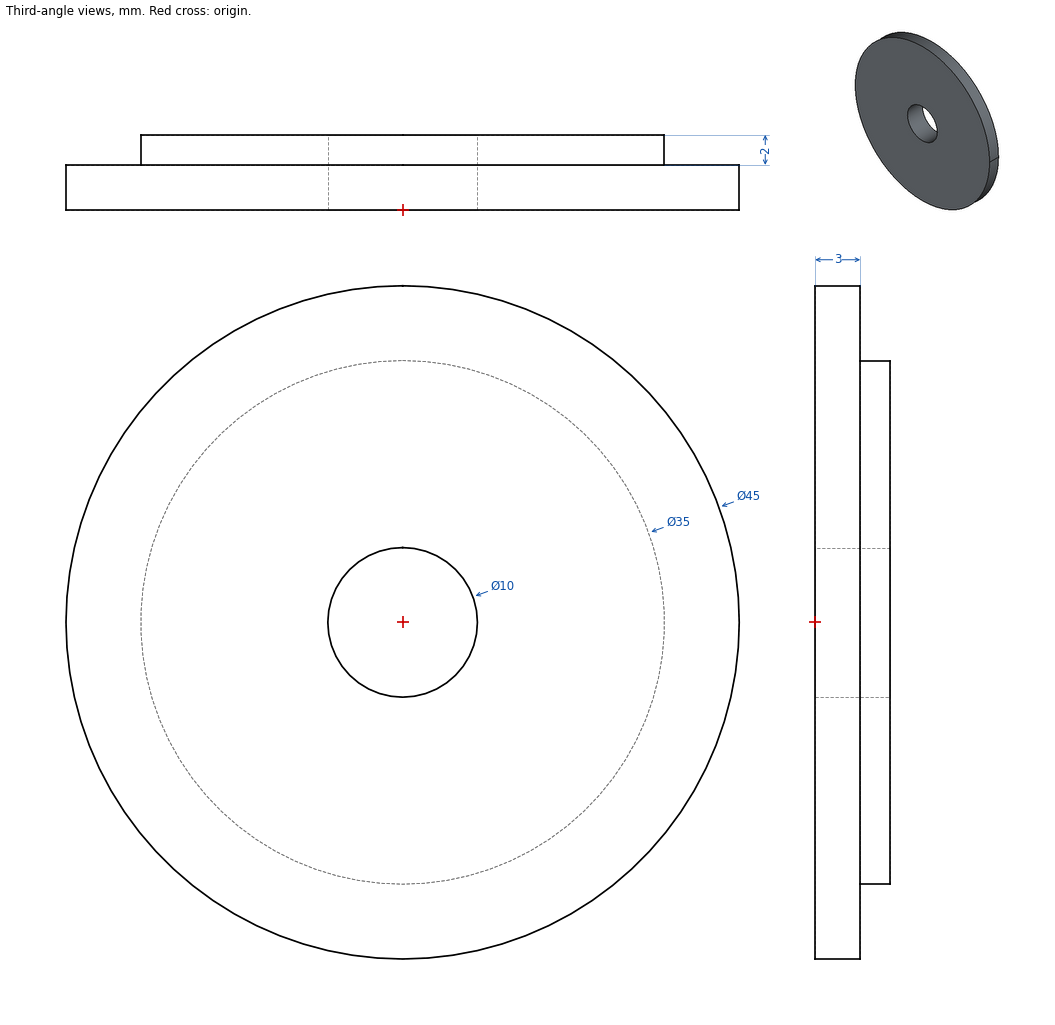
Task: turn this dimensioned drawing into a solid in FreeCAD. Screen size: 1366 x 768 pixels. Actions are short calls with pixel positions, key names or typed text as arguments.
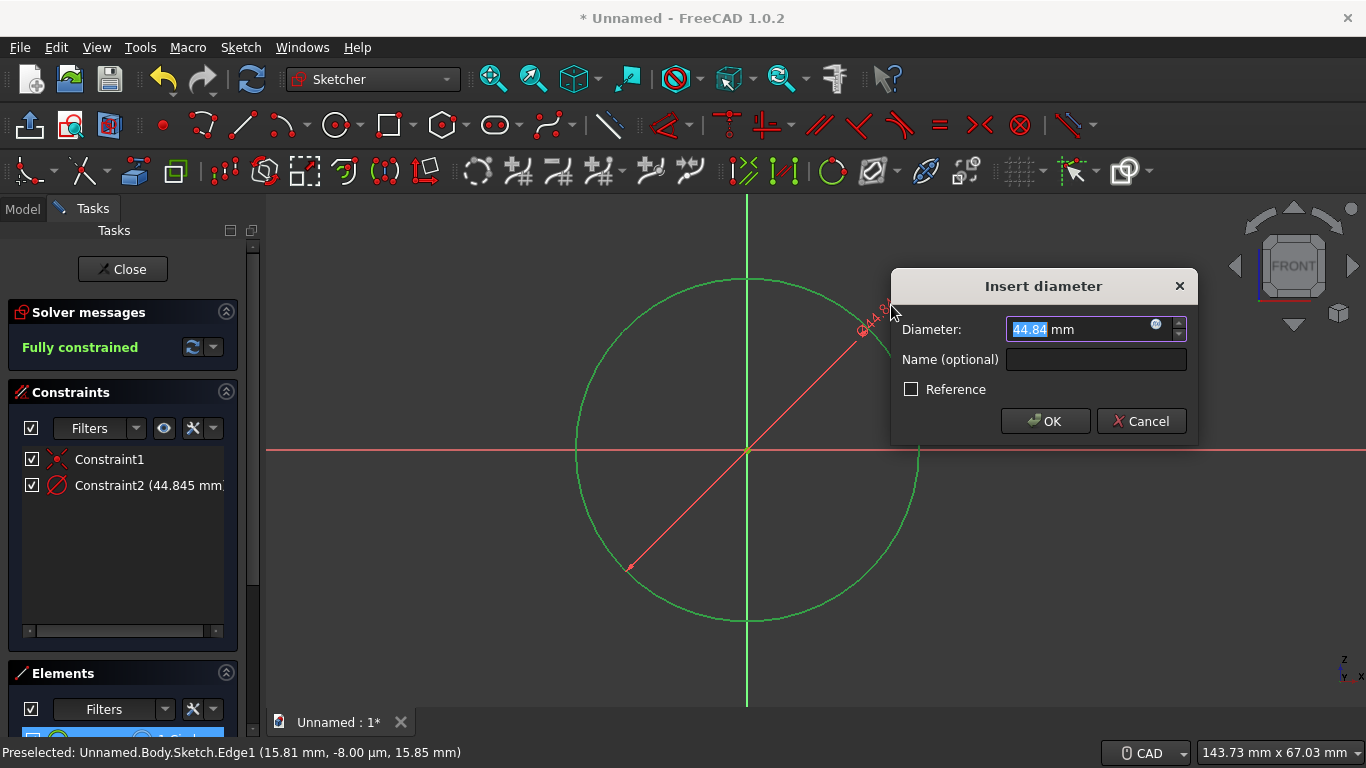
text(45)
key(Return)
key(Escape)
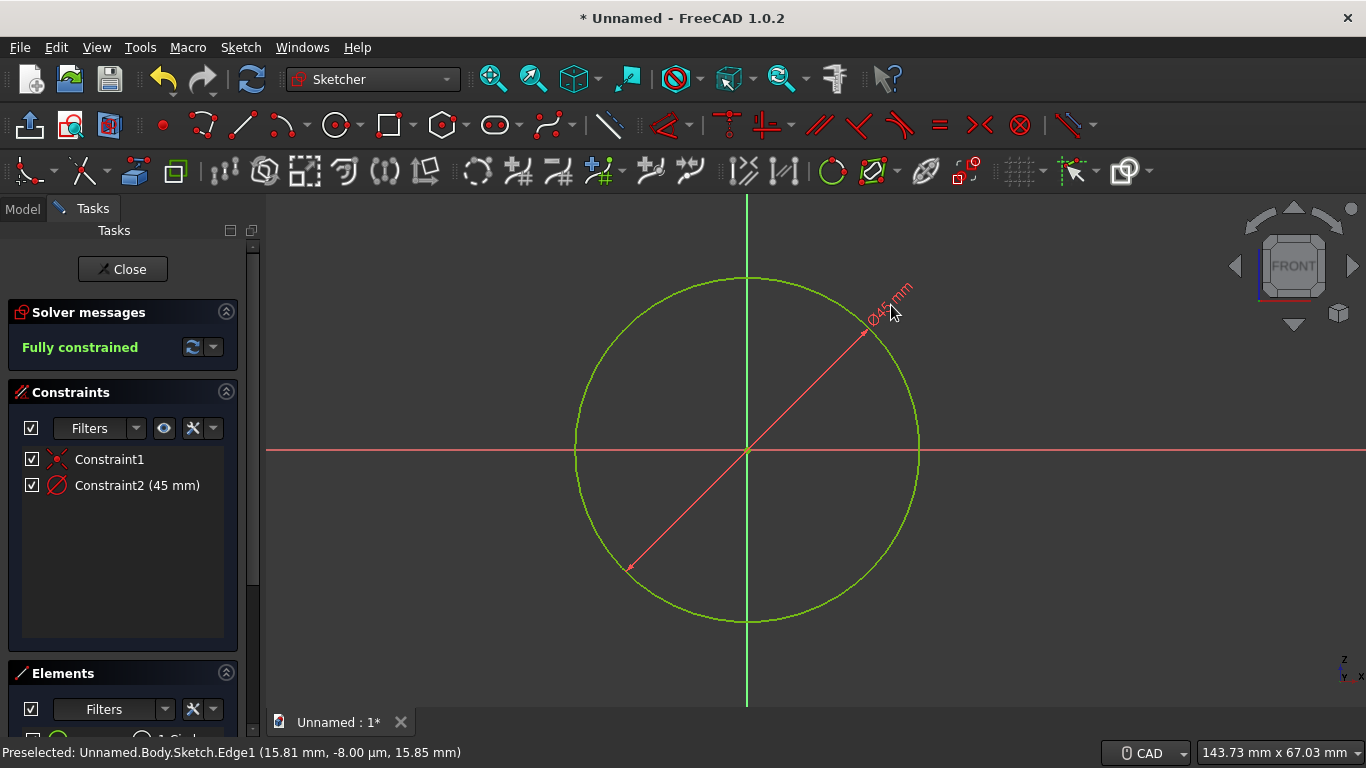
click(123, 269)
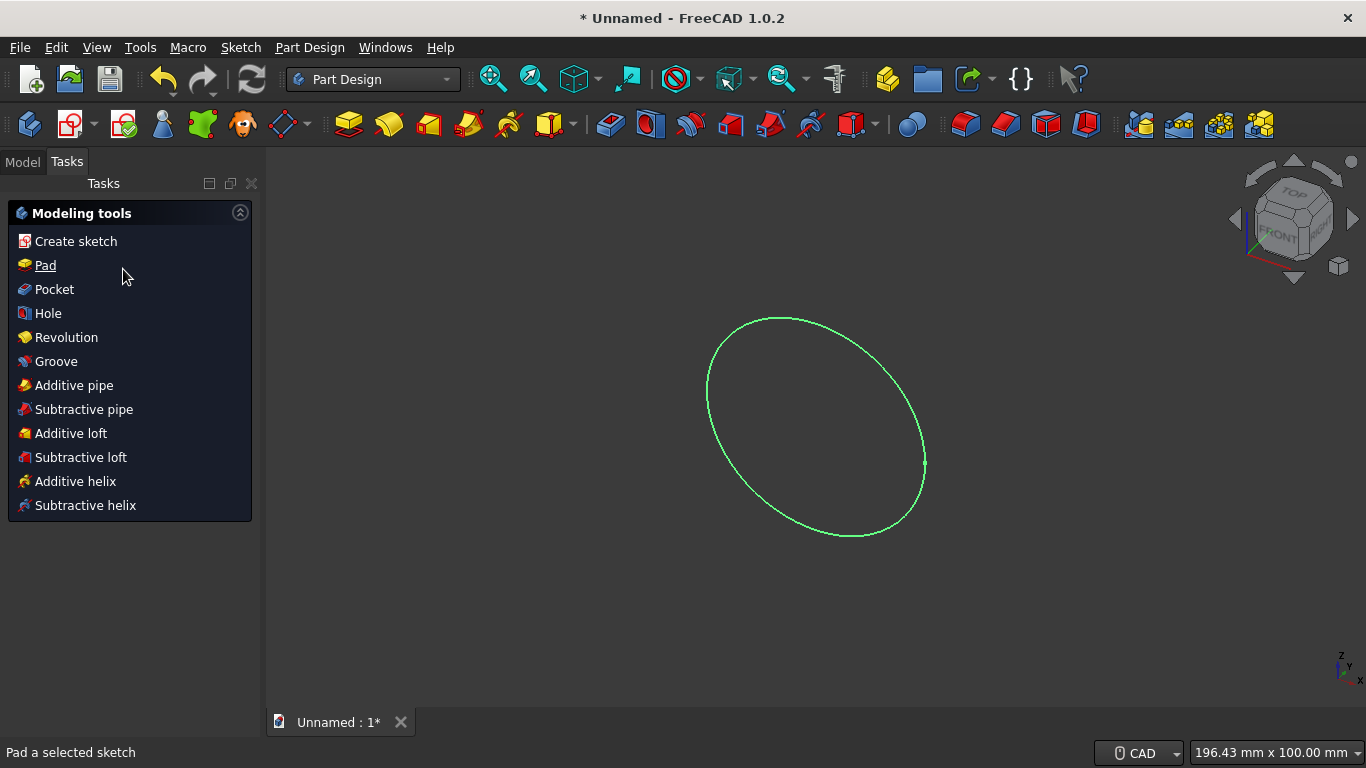
click(350, 124)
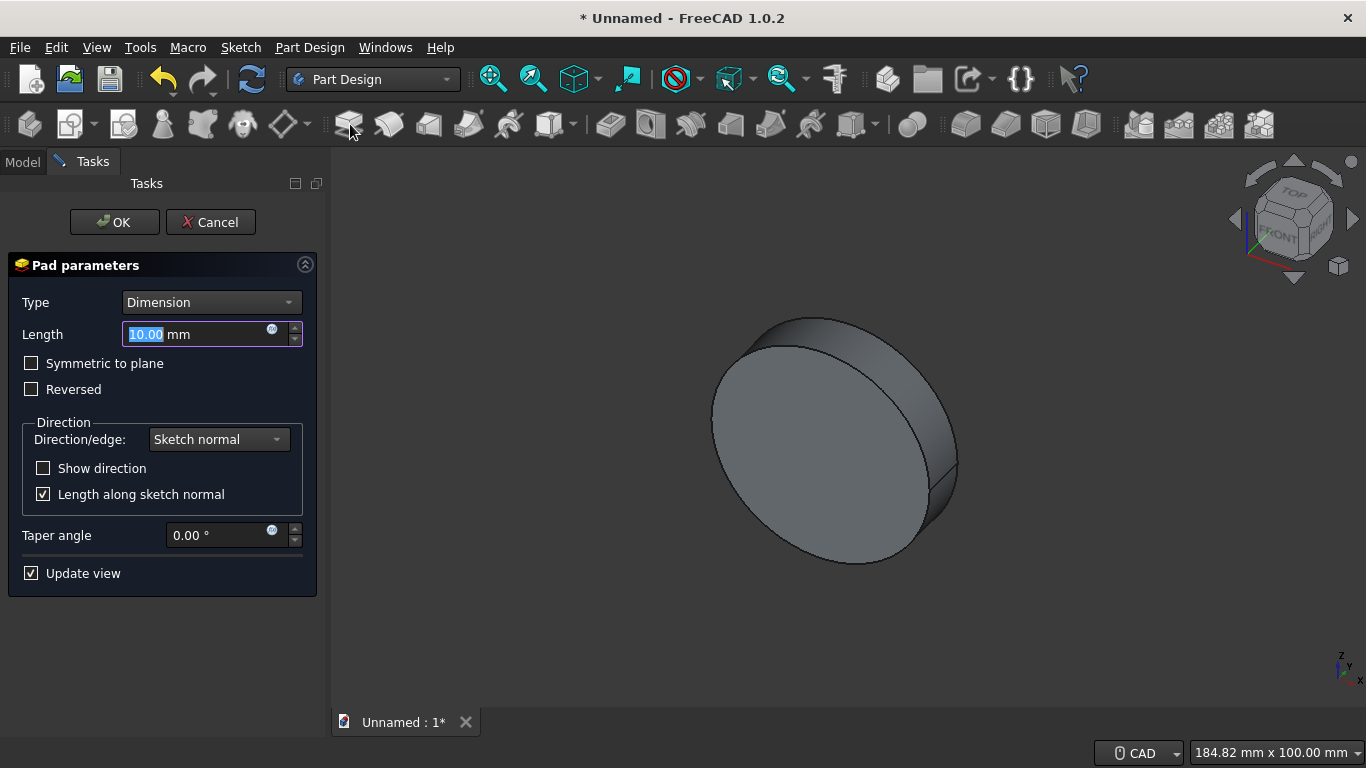
text(3)
key(Tab)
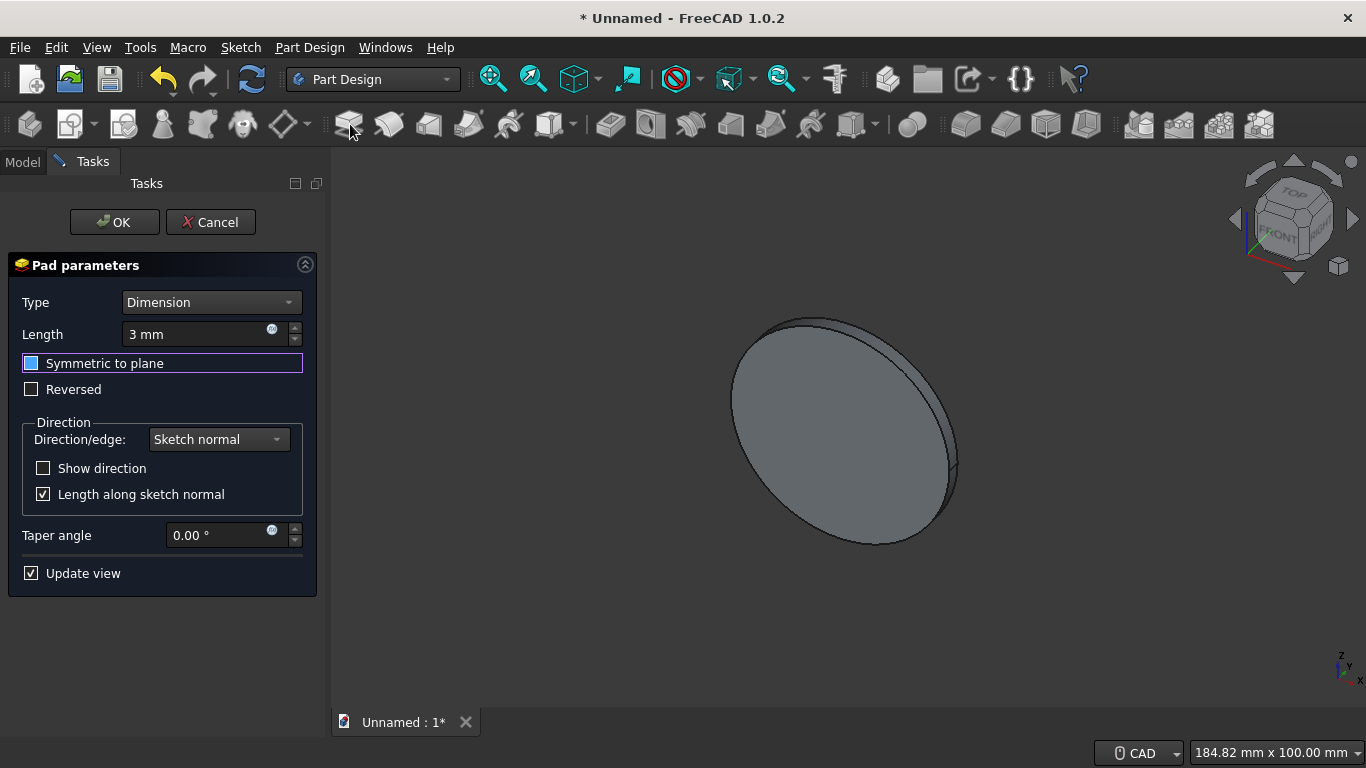
click(30, 389)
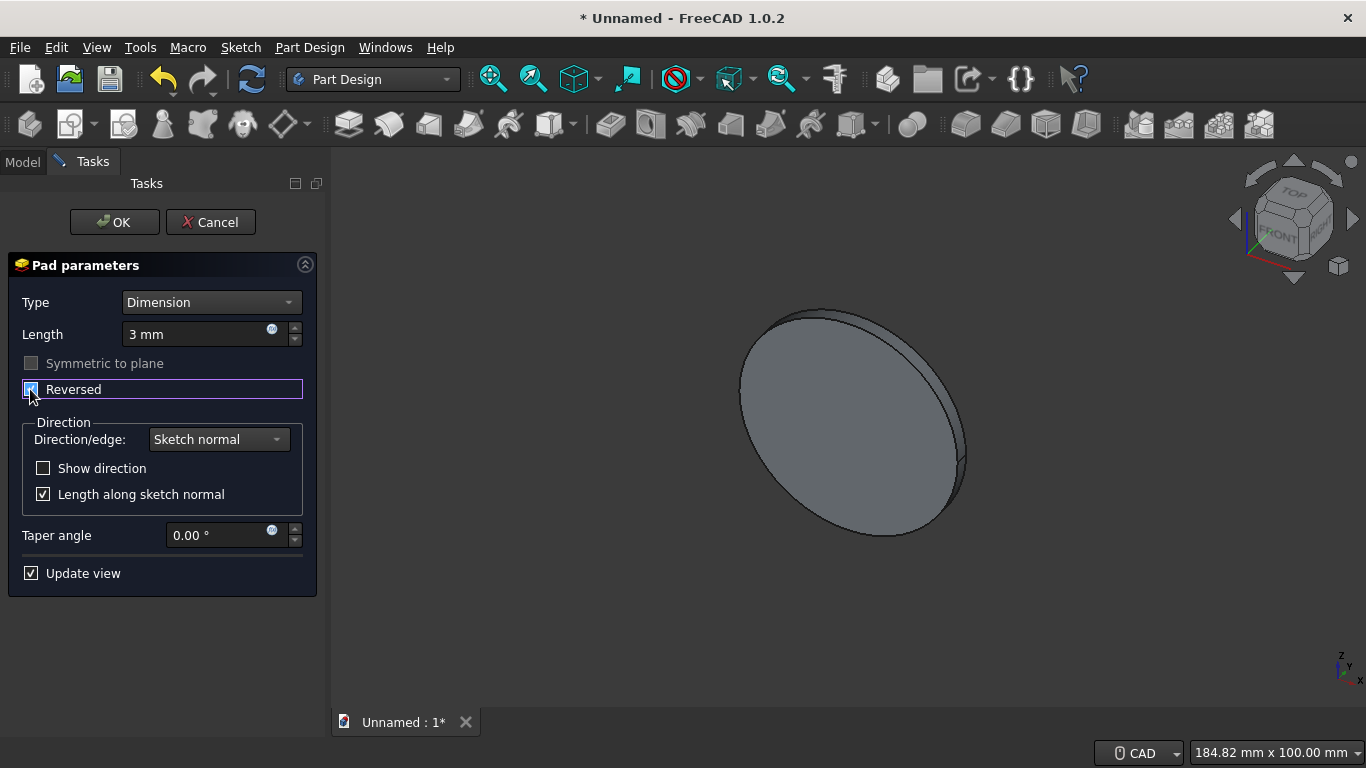
click(115, 222)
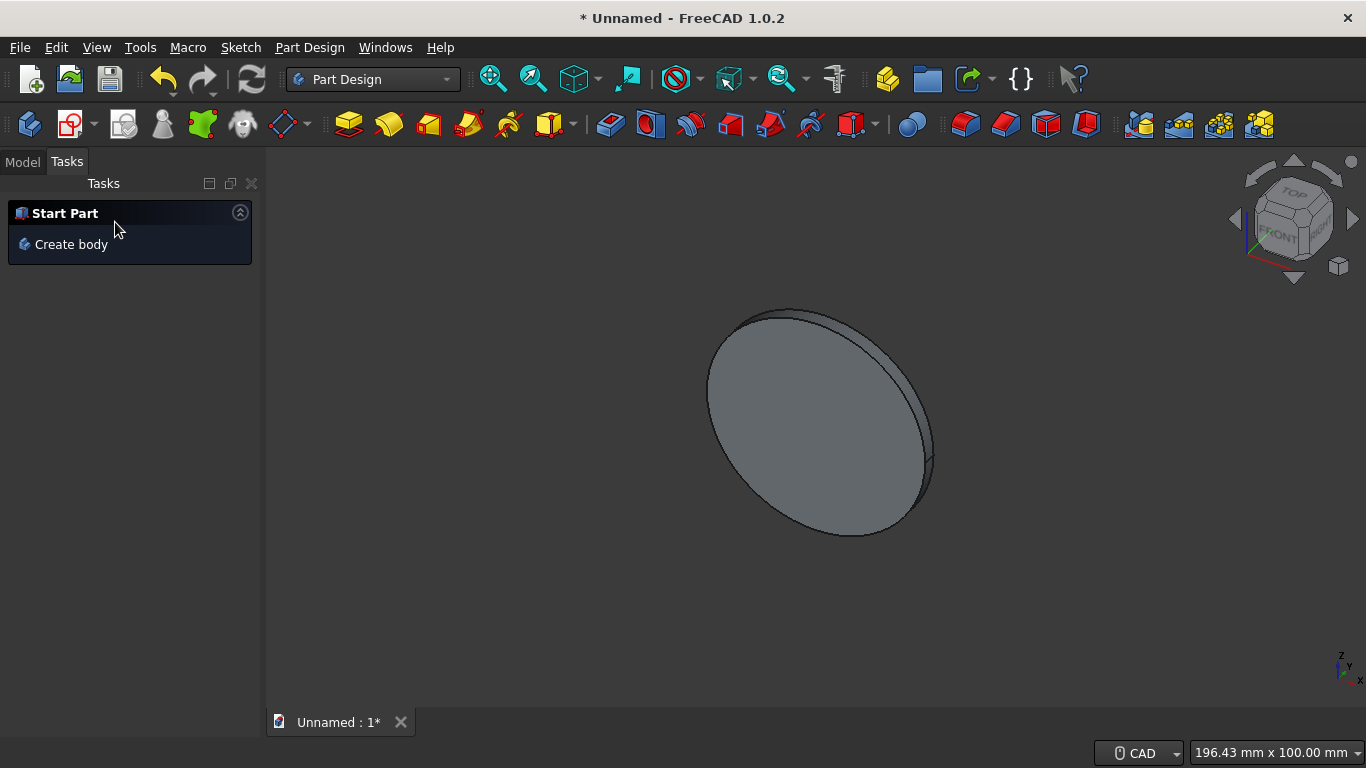
key(4)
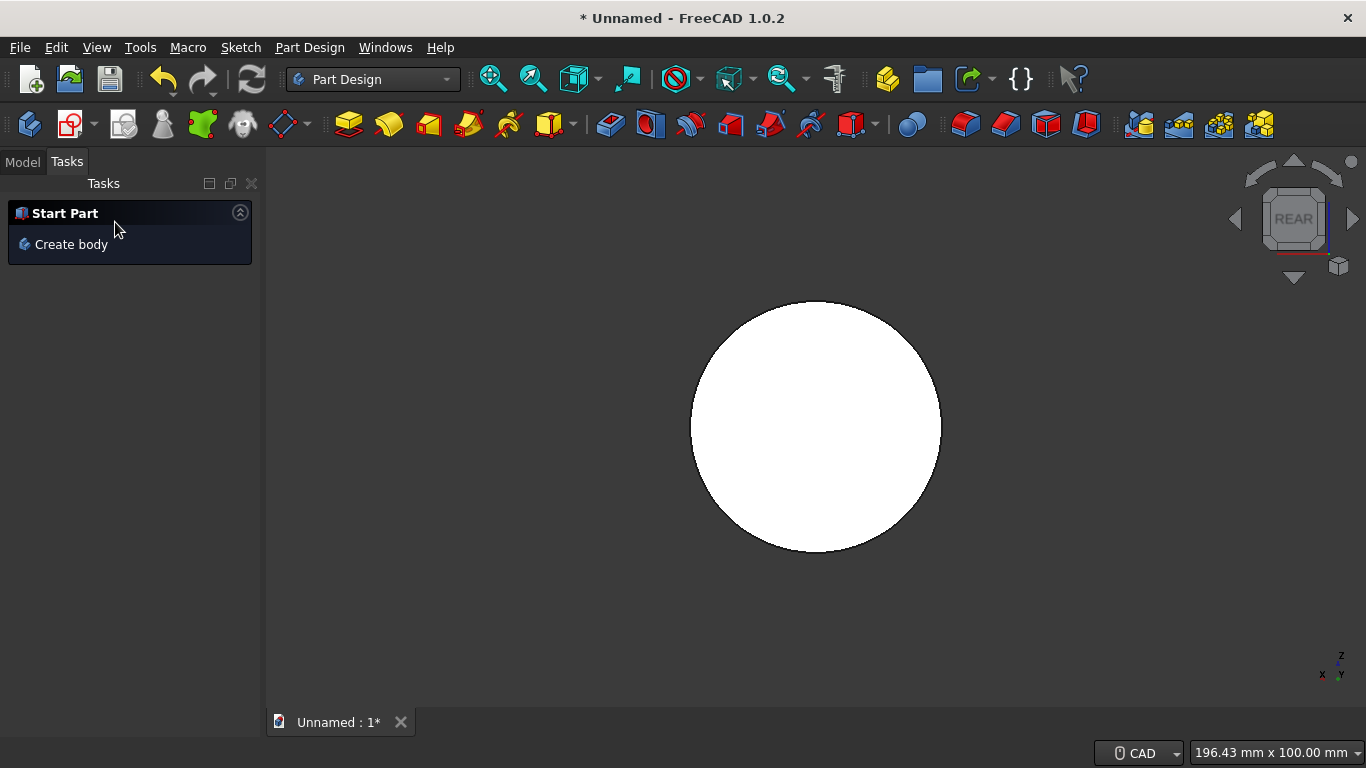
click(816, 426)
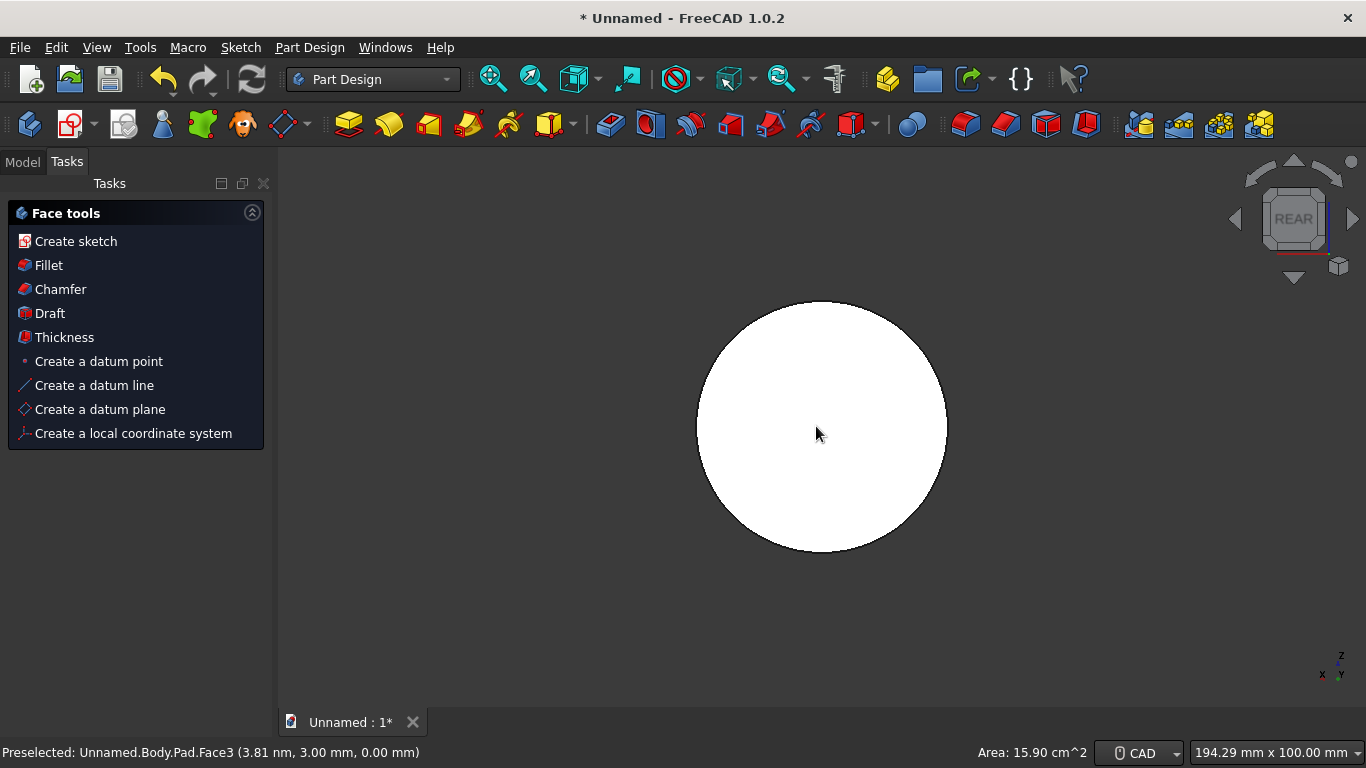
click(70, 124)